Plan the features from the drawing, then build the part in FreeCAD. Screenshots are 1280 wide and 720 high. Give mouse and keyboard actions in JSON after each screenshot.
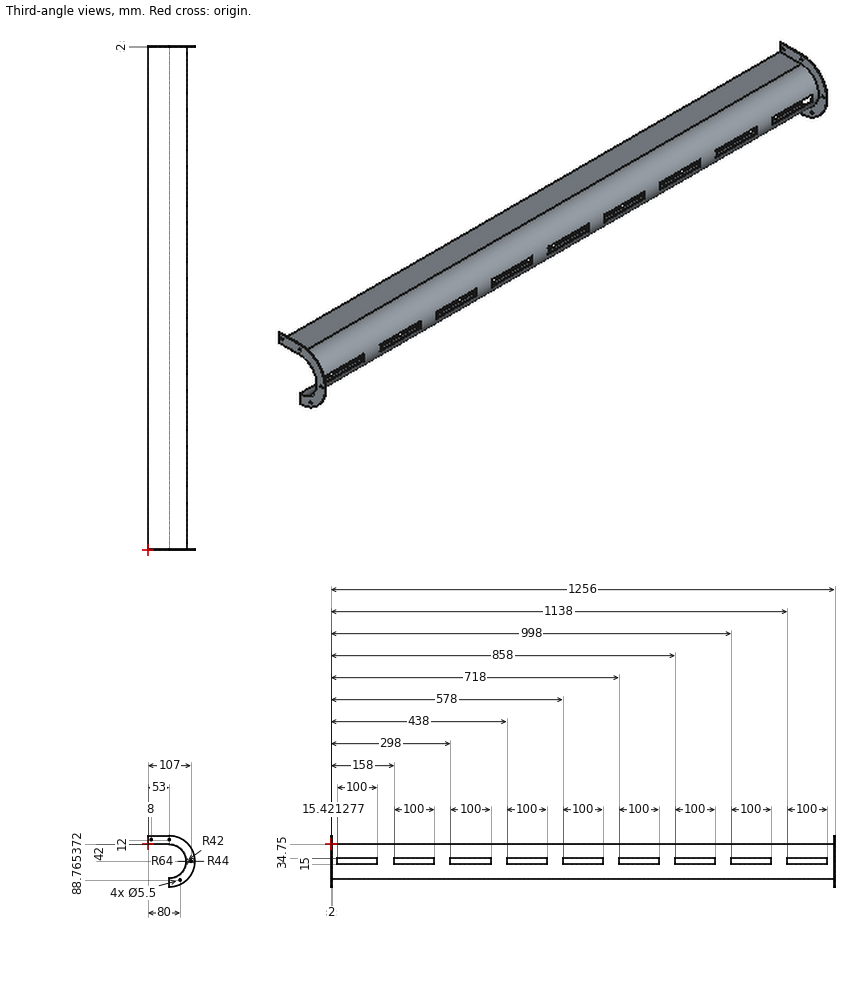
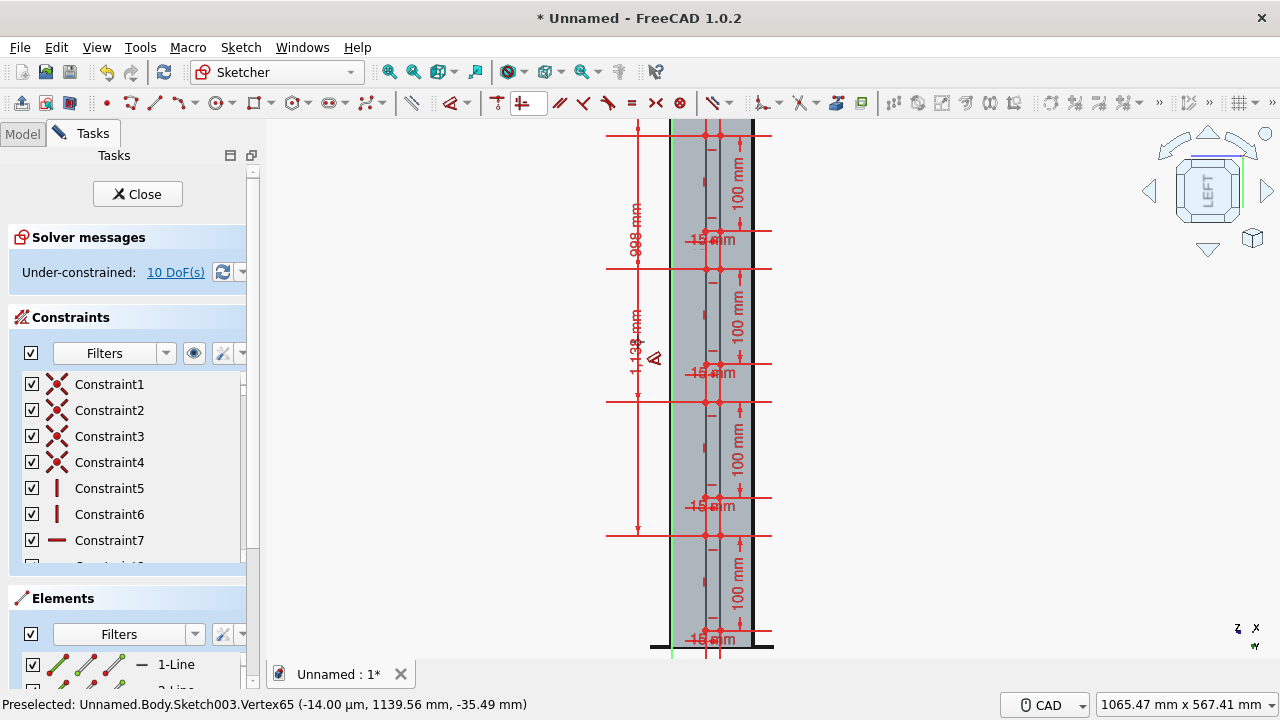
{"action": "scroll", "coordinate": [708, 539], "scroll_direction": "down", "scroll_amount": 6}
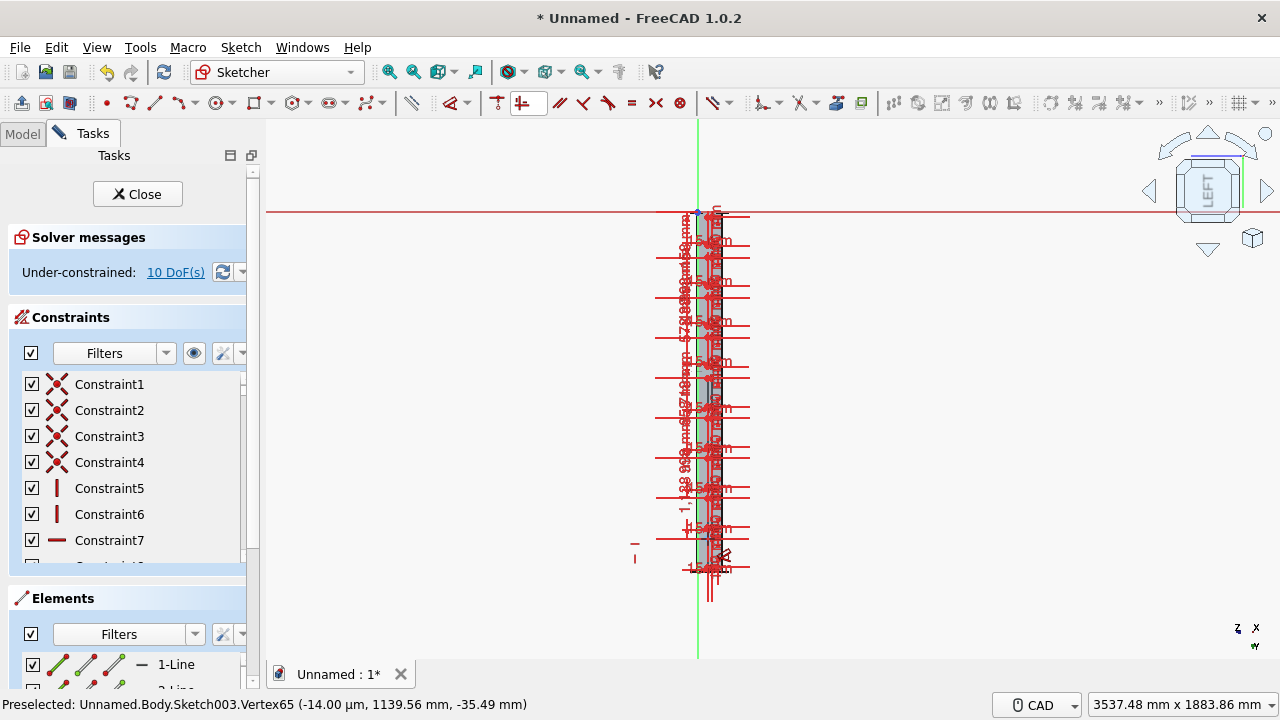
{"action": "scroll", "coordinate": [708, 217], "scroll_direction": "up", "scroll_amount": 7}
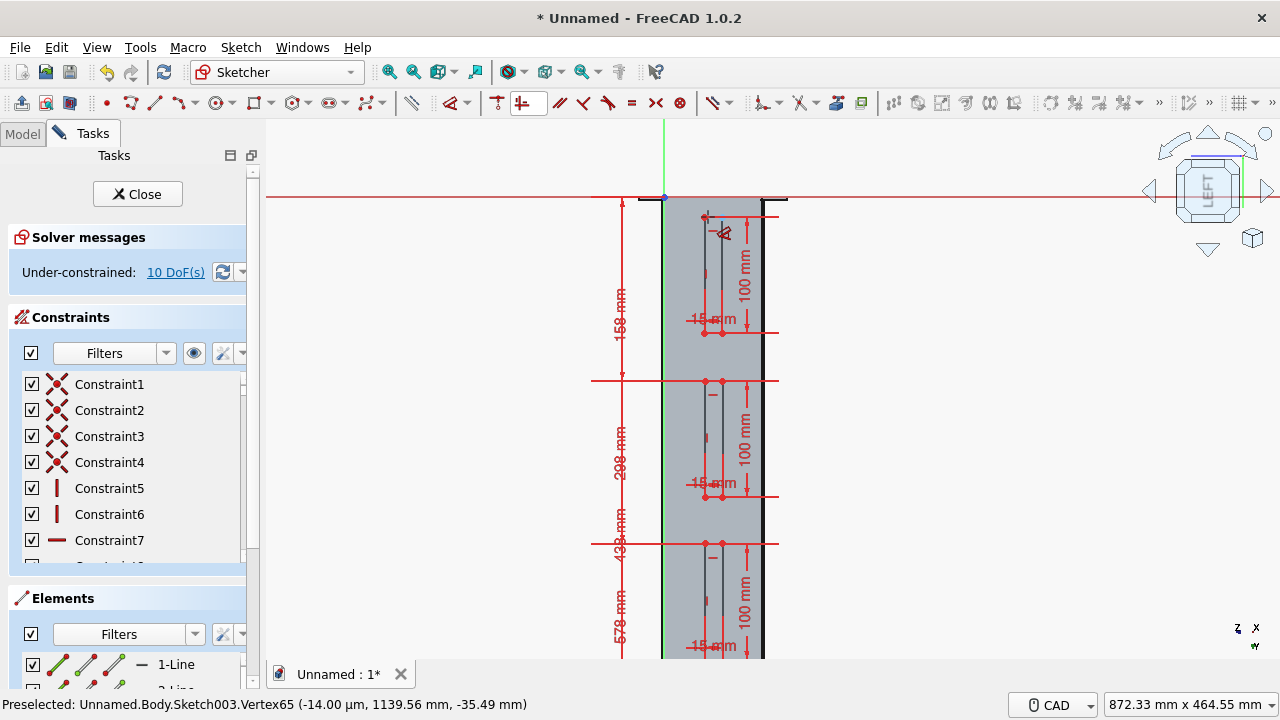
{"action": "left_click", "coordinate": [705, 217]}
{"action": "left_click", "coordinate": [685, 163]}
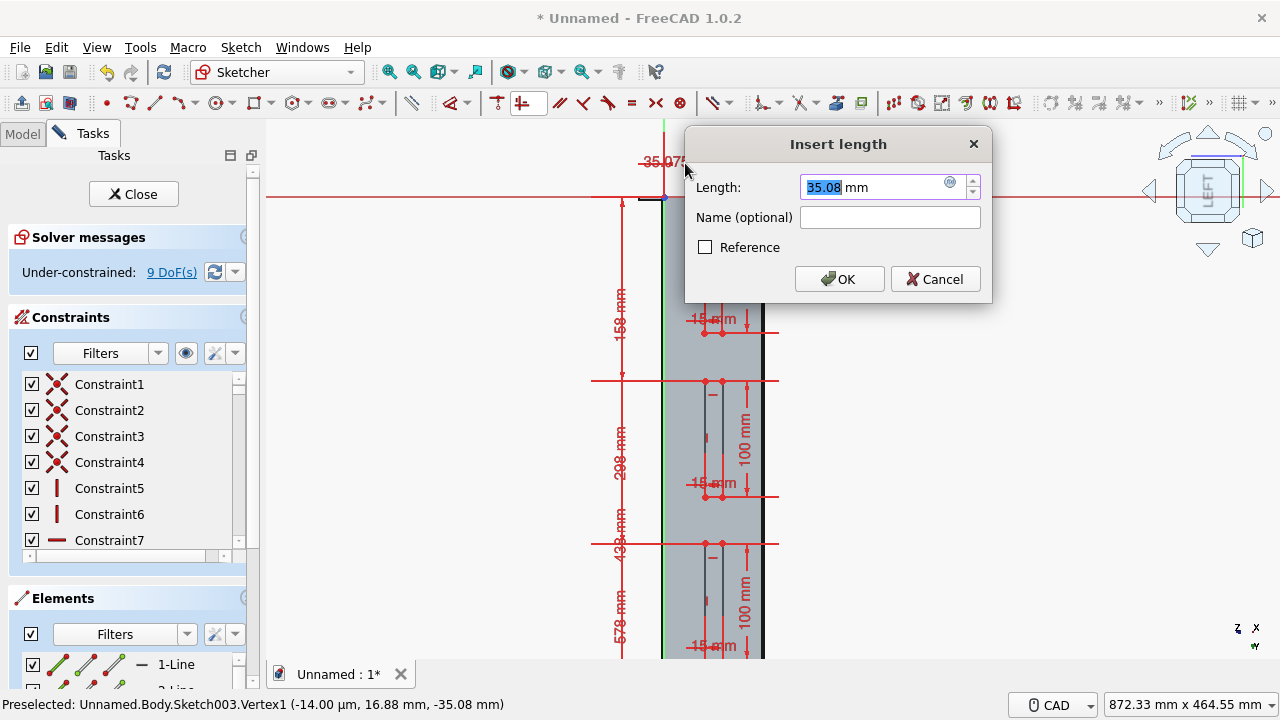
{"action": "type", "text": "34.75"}
{"action": "key", "text": "Return"}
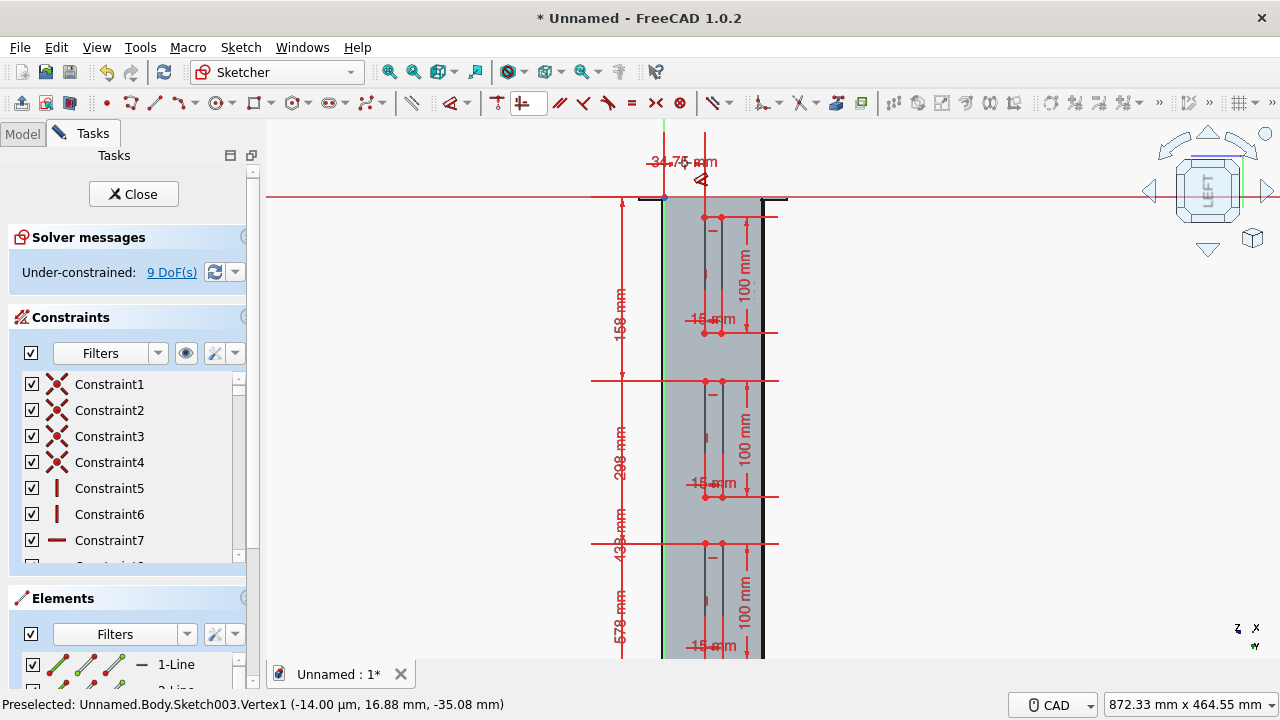
{"action": "left_click", "coordinate": [705, 381]}
{"action": "left_click", "coordinate": [685, 415]}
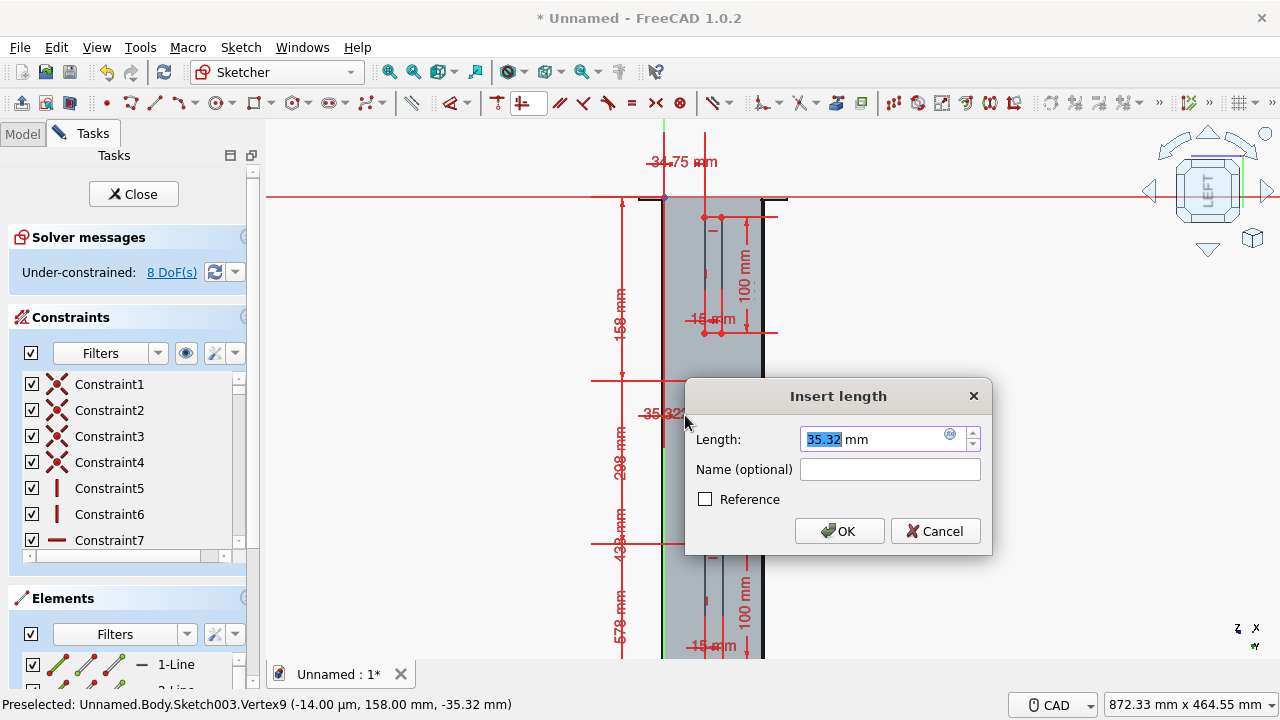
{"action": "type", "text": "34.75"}
{"action": "key", "text": "Return"}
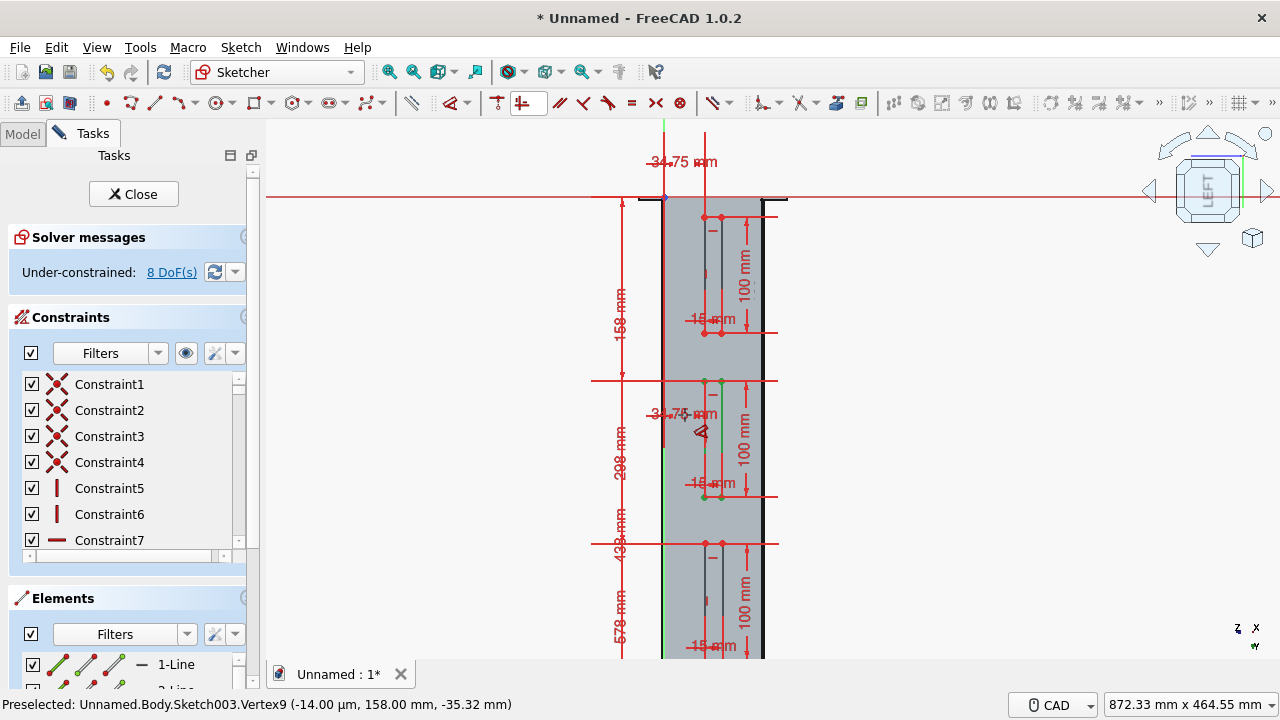
{"action": "scroll", "coordinate": [708, 216], "scroll_direction": "down", "scroll_amount": 7}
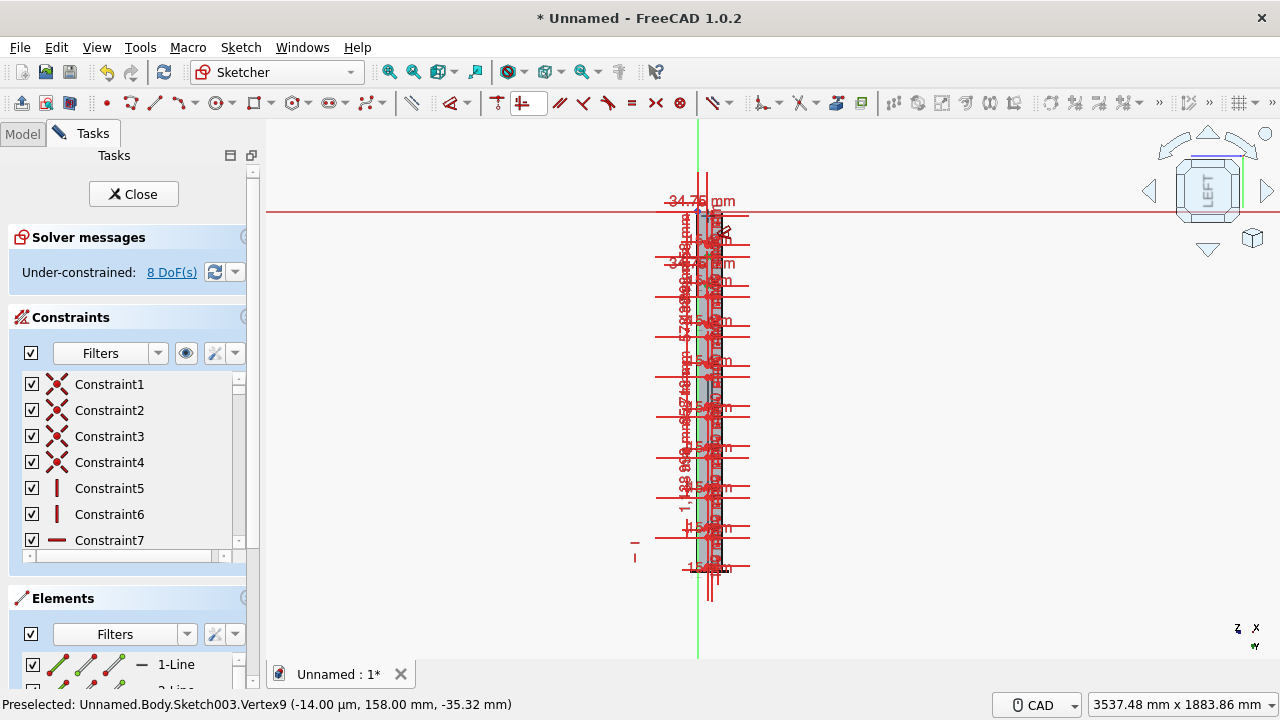
{"action": "scroll", "coordinate": [708, 498], "scroll_direction": "up", "scroll_amount": 7}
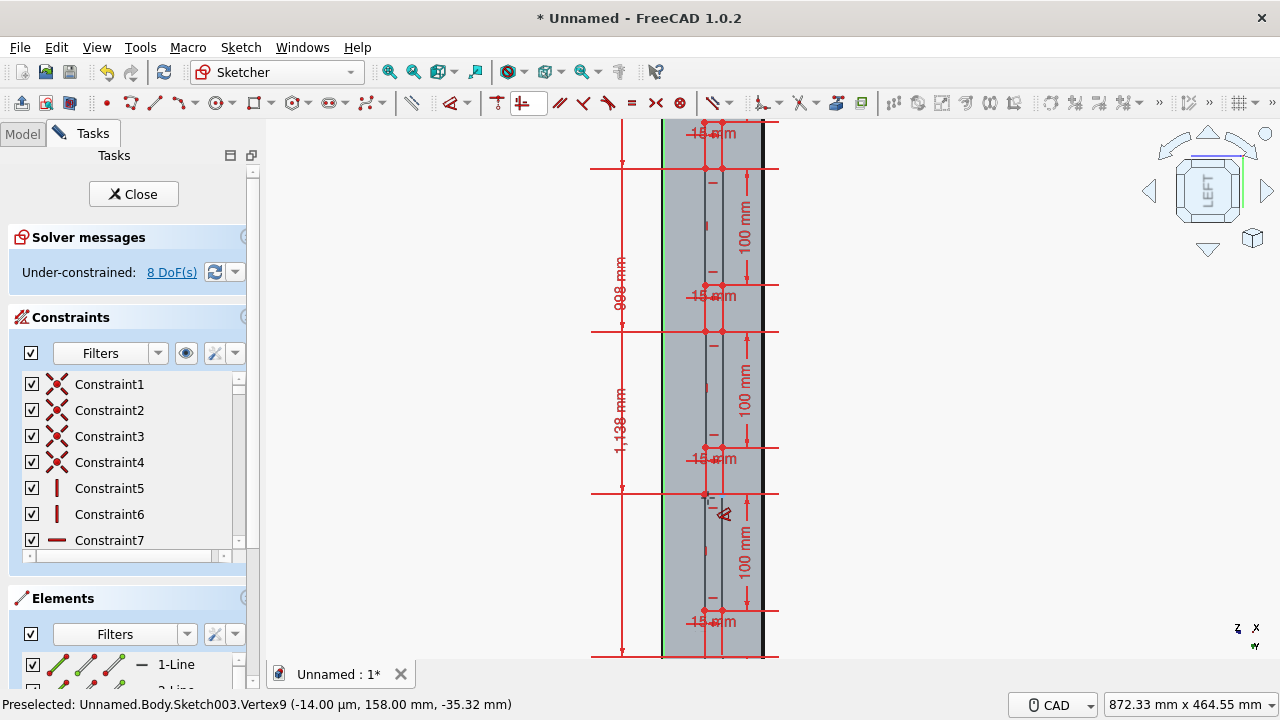
{"action": "left_click", "coordinate": [705, 494]}
{"action": "left_click", "coordinate": [685, 528]}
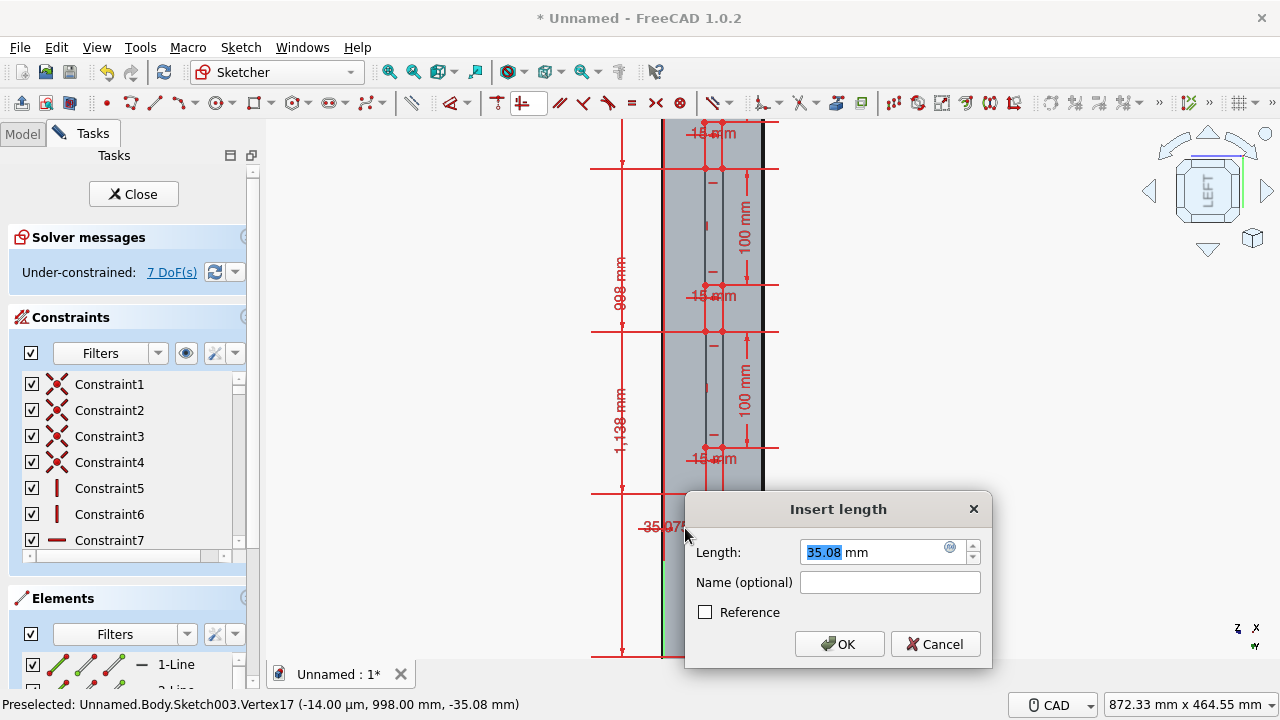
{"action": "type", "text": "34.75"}
{"action": "key", "text": "Return"}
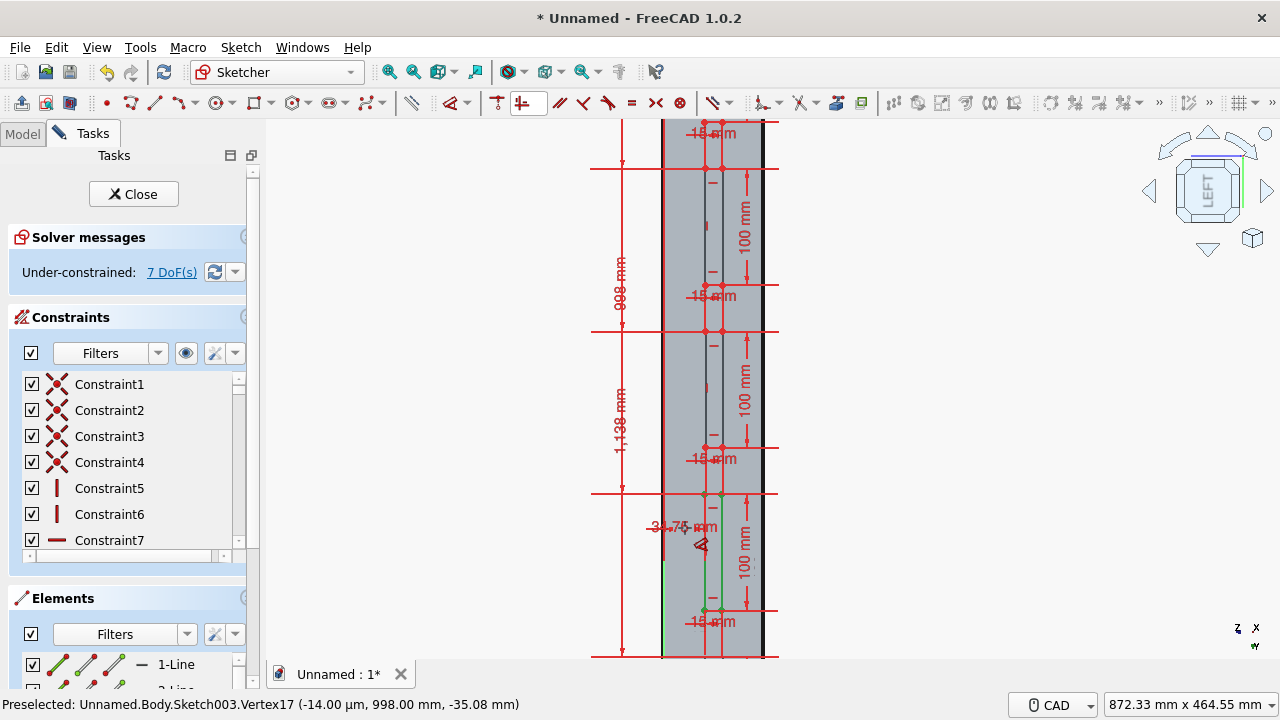
{"action": "scroll", "coordinate": [708, 499], "scroll_direction": "down", "scroll_amount": 7}